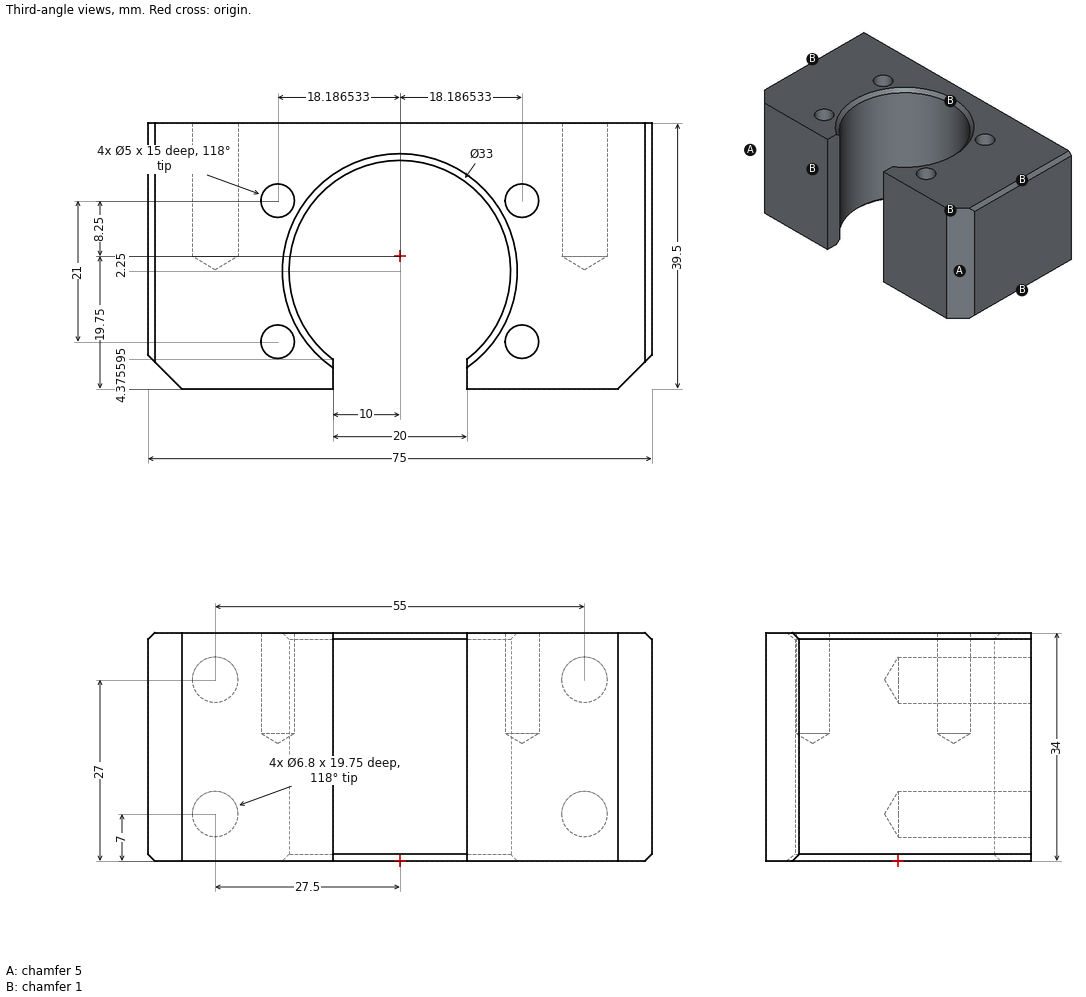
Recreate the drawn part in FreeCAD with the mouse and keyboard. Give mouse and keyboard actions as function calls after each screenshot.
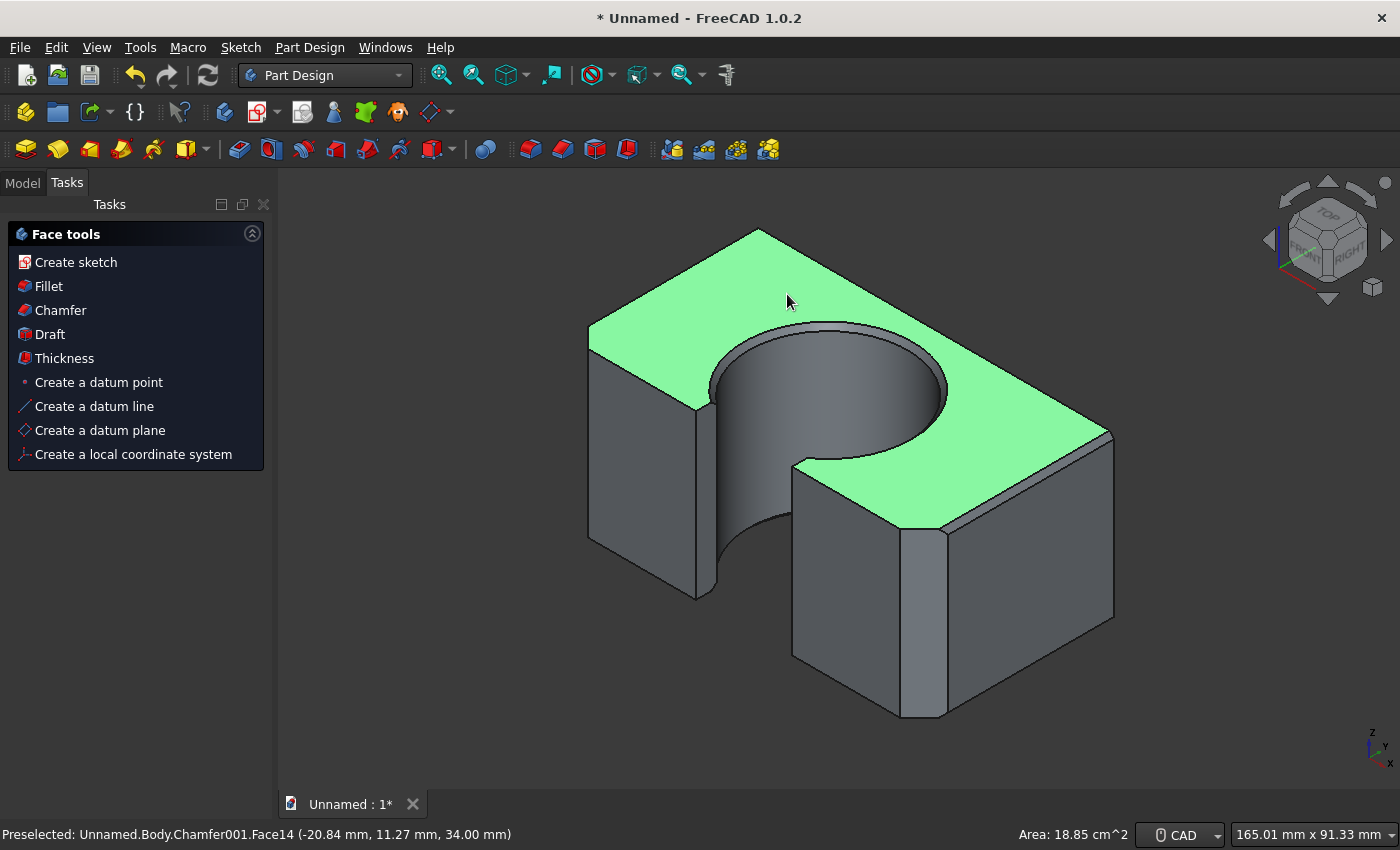
click(258, 112)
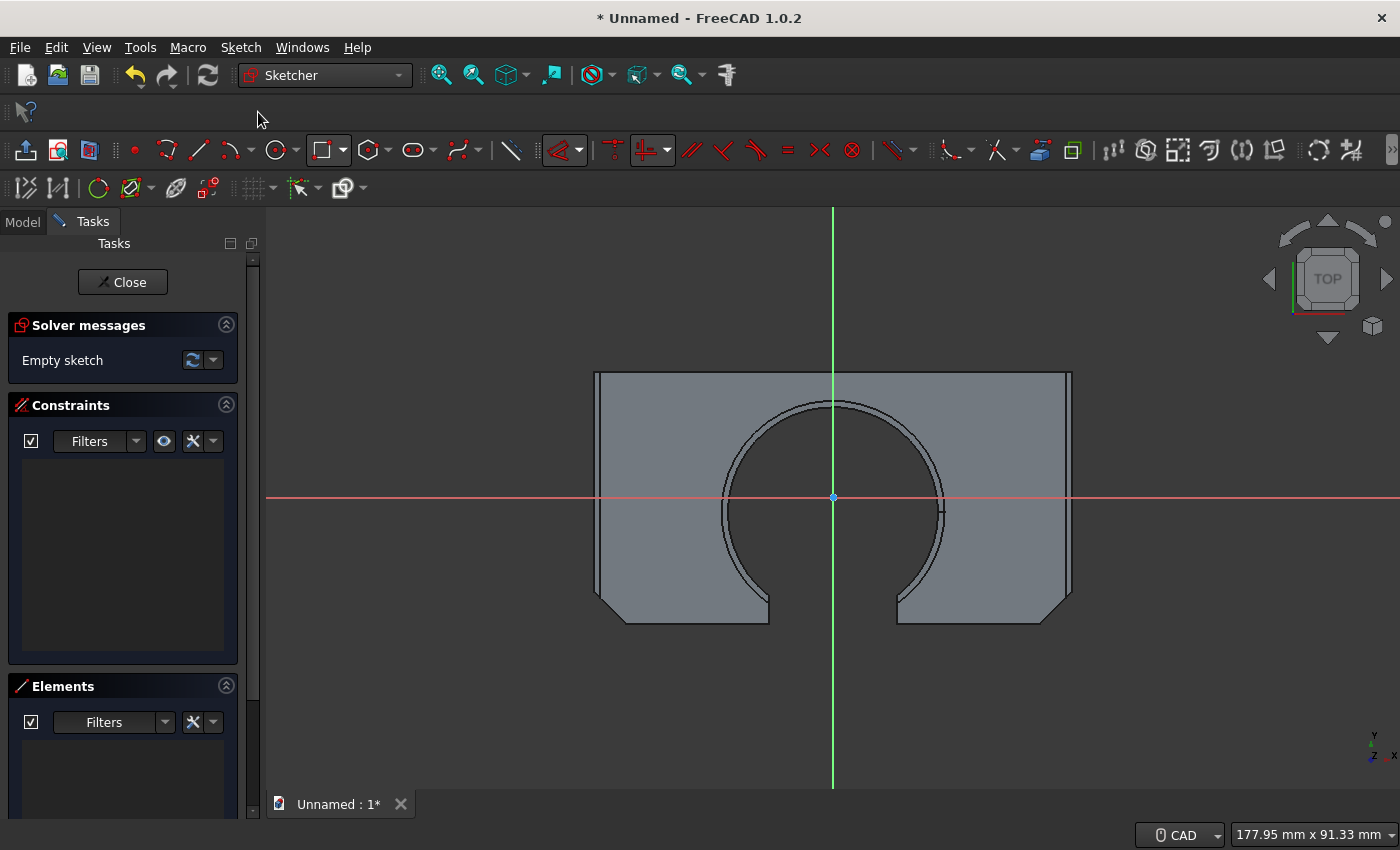
scroll(889, 524, up, 4)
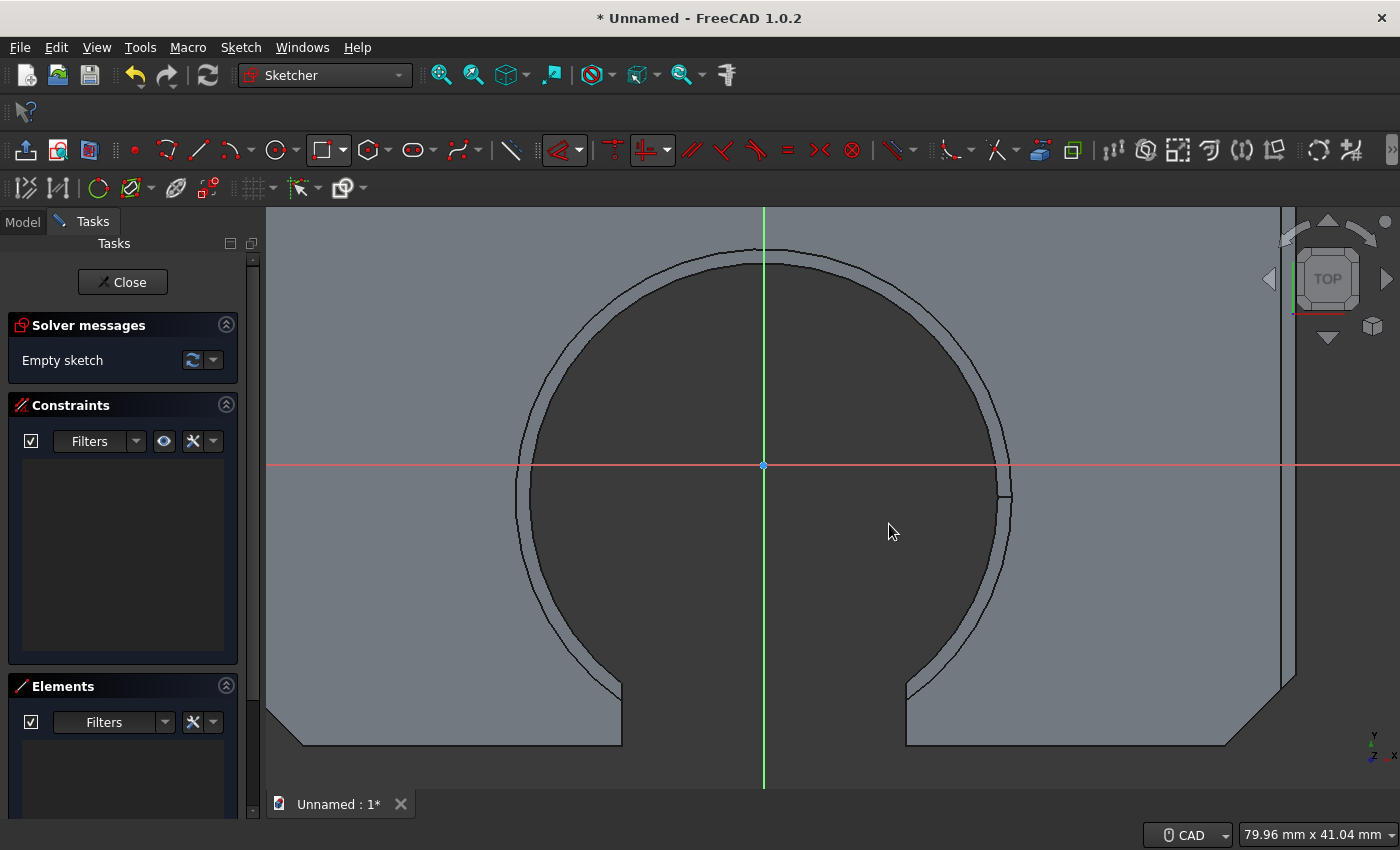
key(g)
key(c)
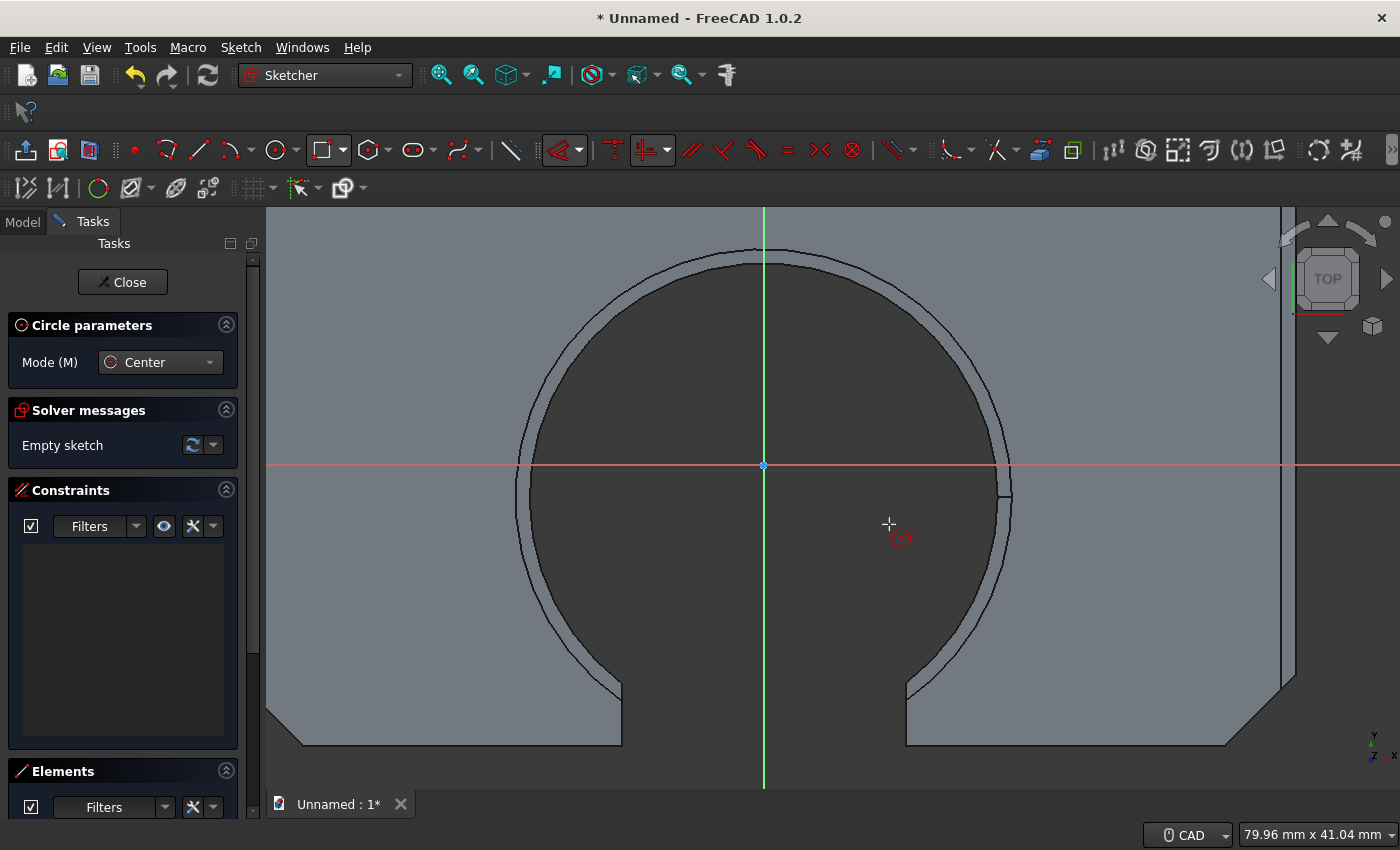
click(506, 348)
click(531, 323)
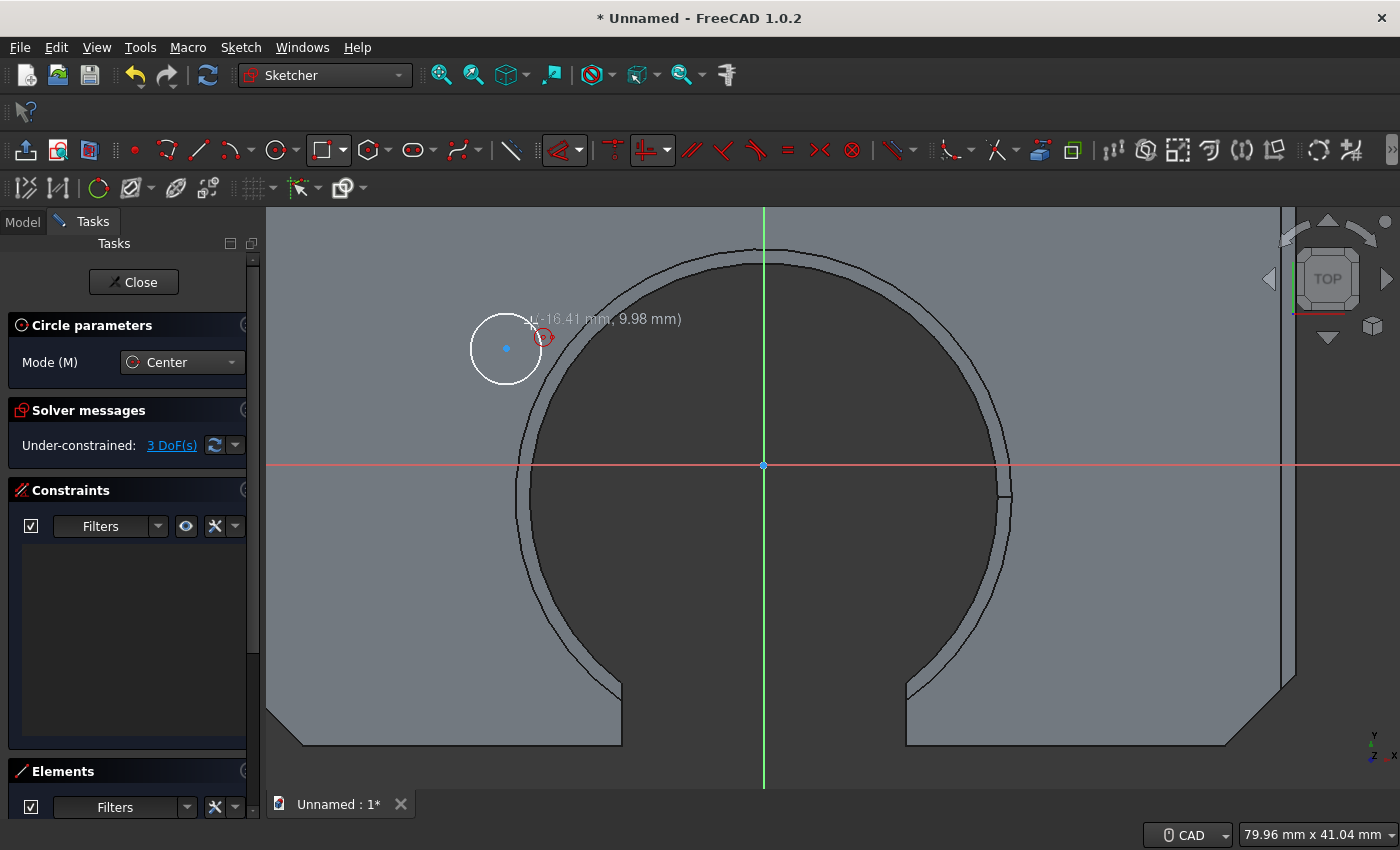
click(506, 646)
click(531, 621)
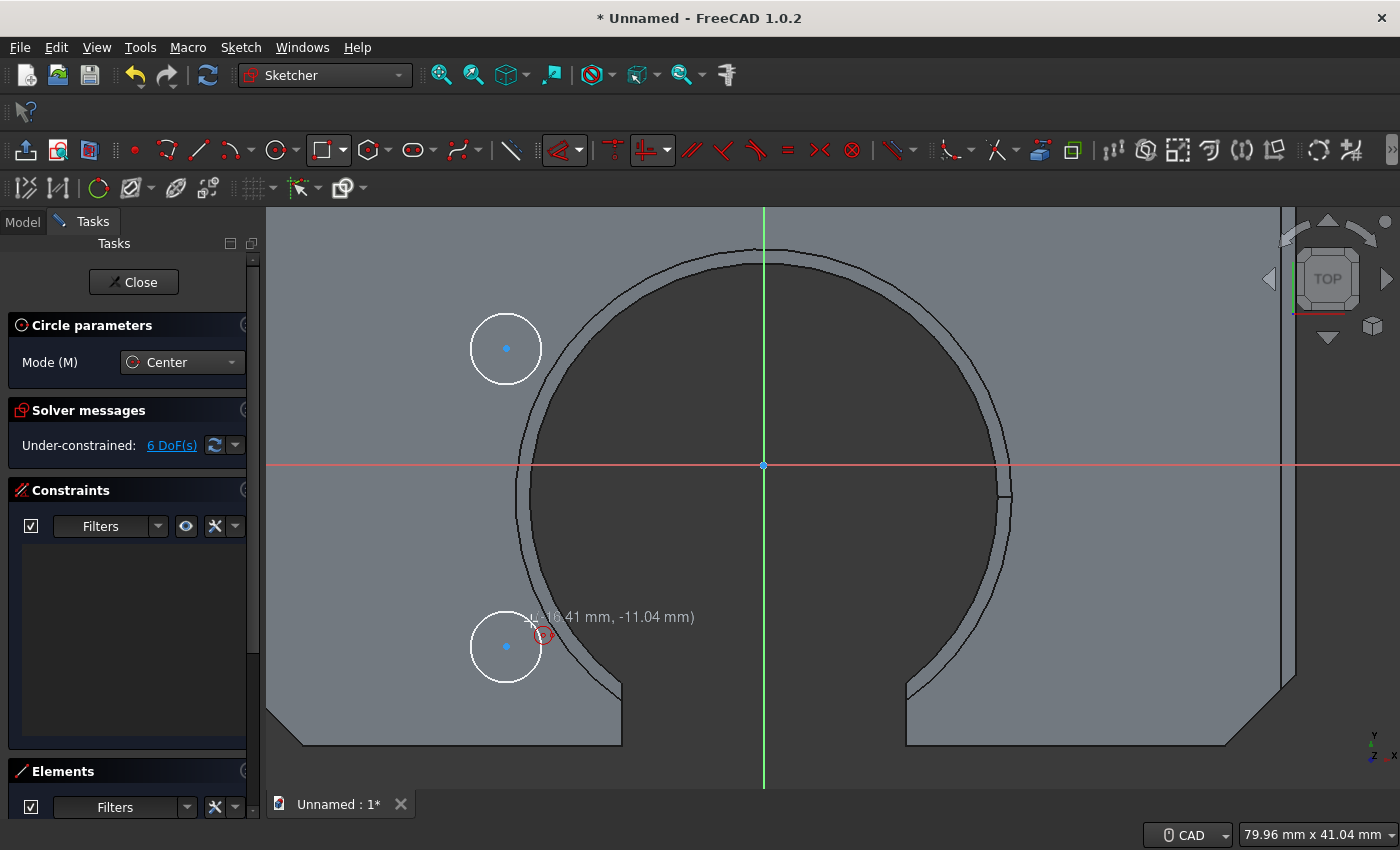
click(1022, 348)
click(1047, 323)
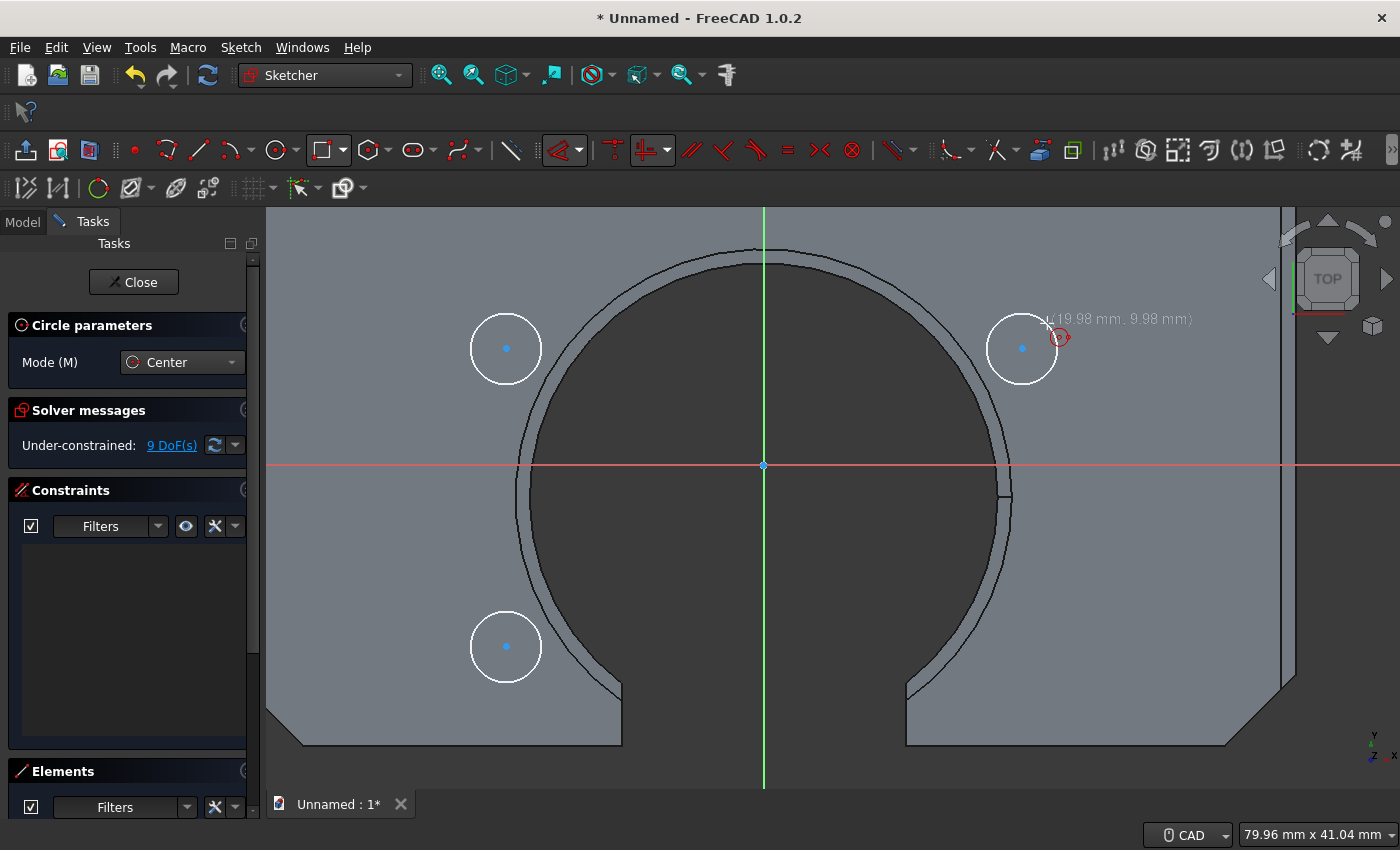
click(1022, 646)
click(1047, 621)
key(Escape)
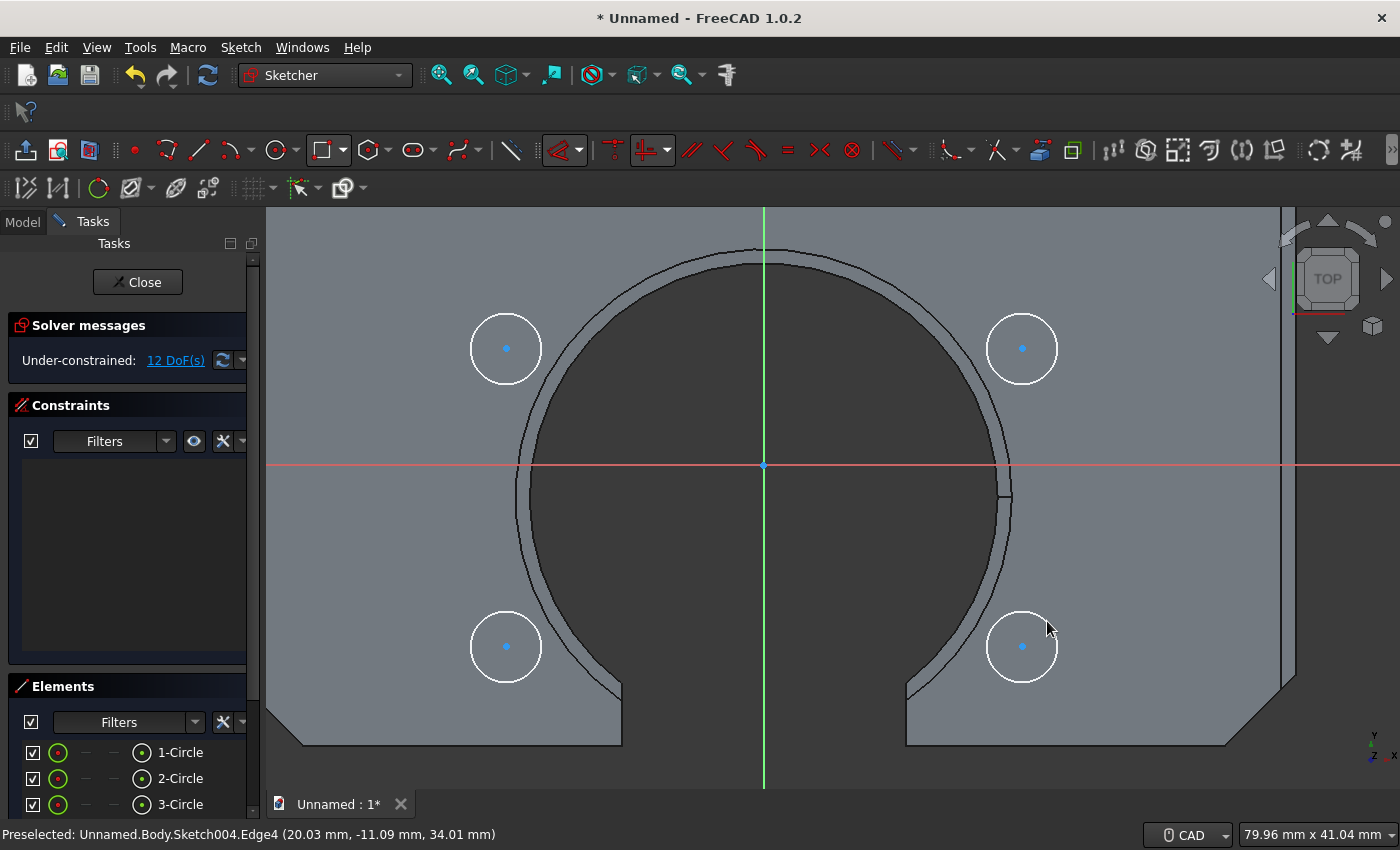
click(531, 324)